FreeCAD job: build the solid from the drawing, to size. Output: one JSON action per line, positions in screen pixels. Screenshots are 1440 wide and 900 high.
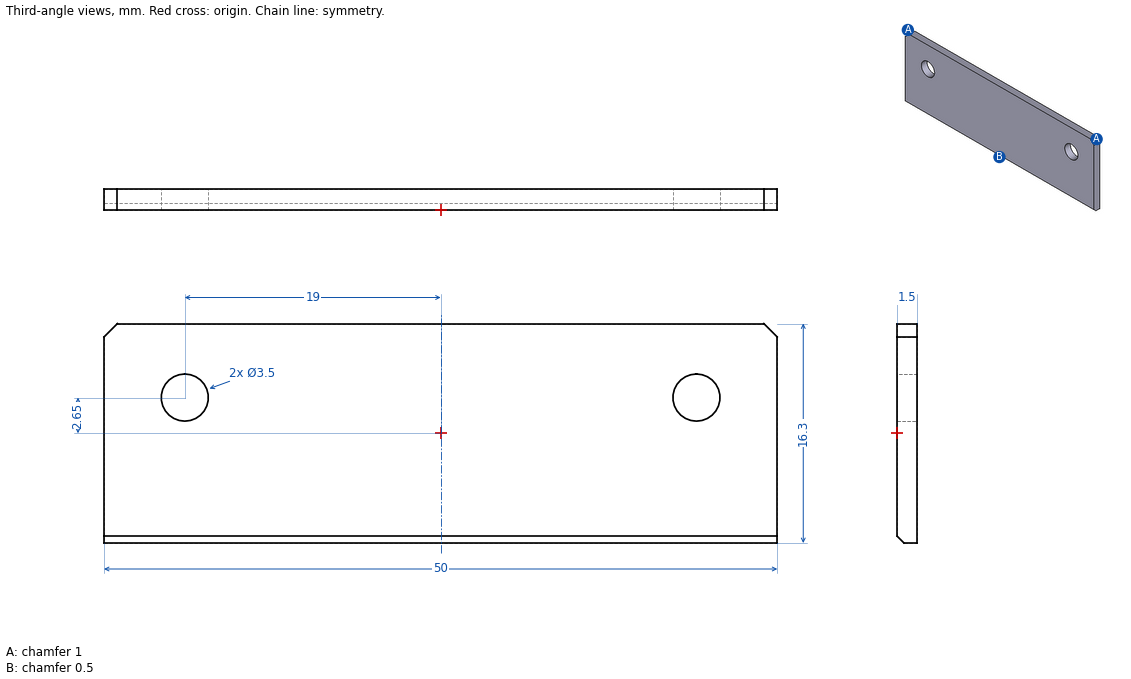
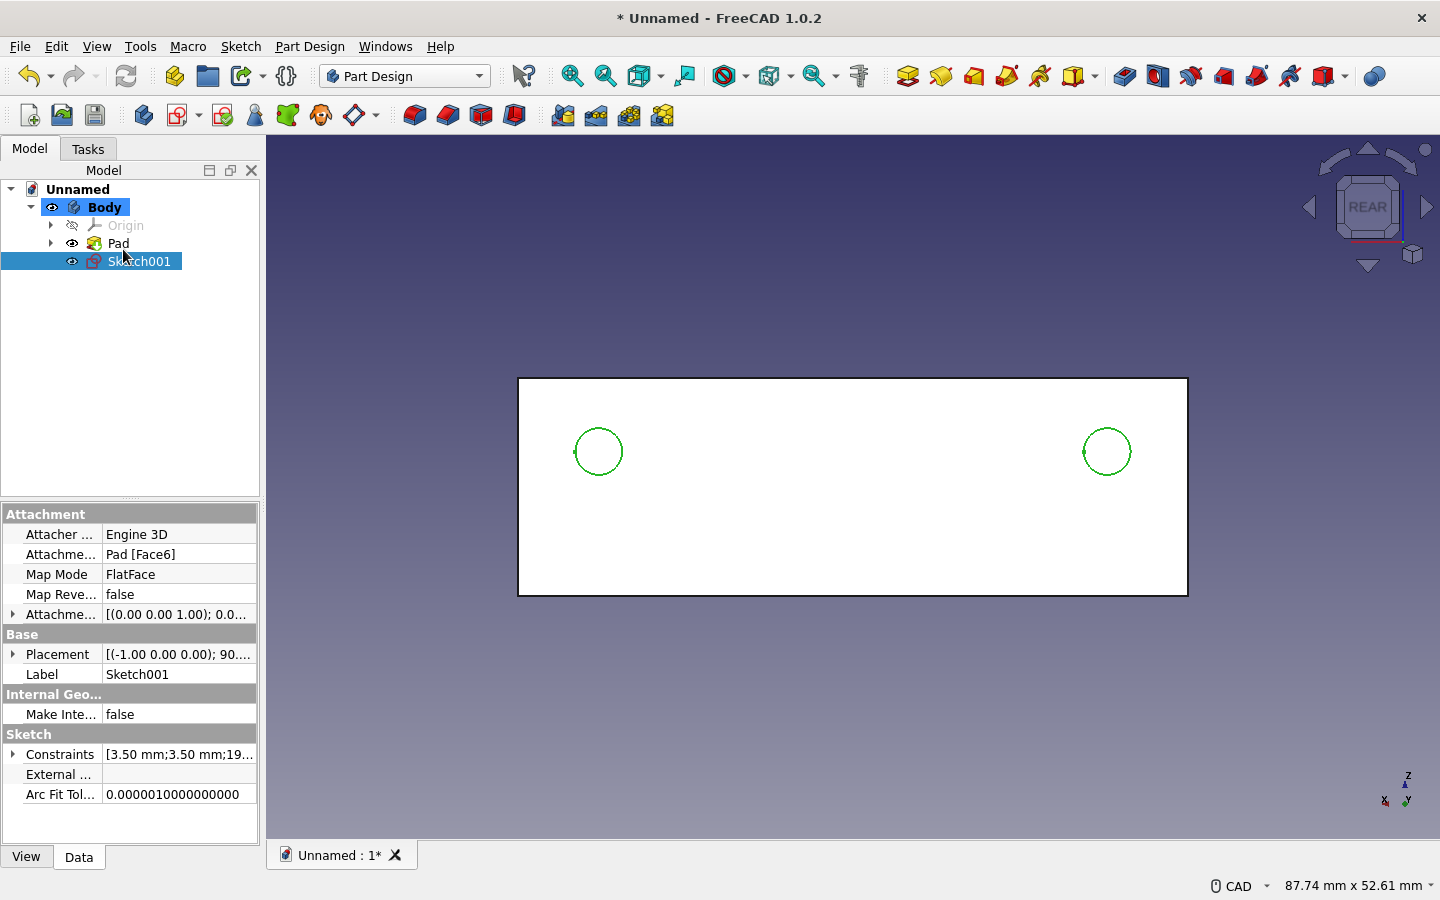
{"action": "left_click", "coordinate": [1125, 76]}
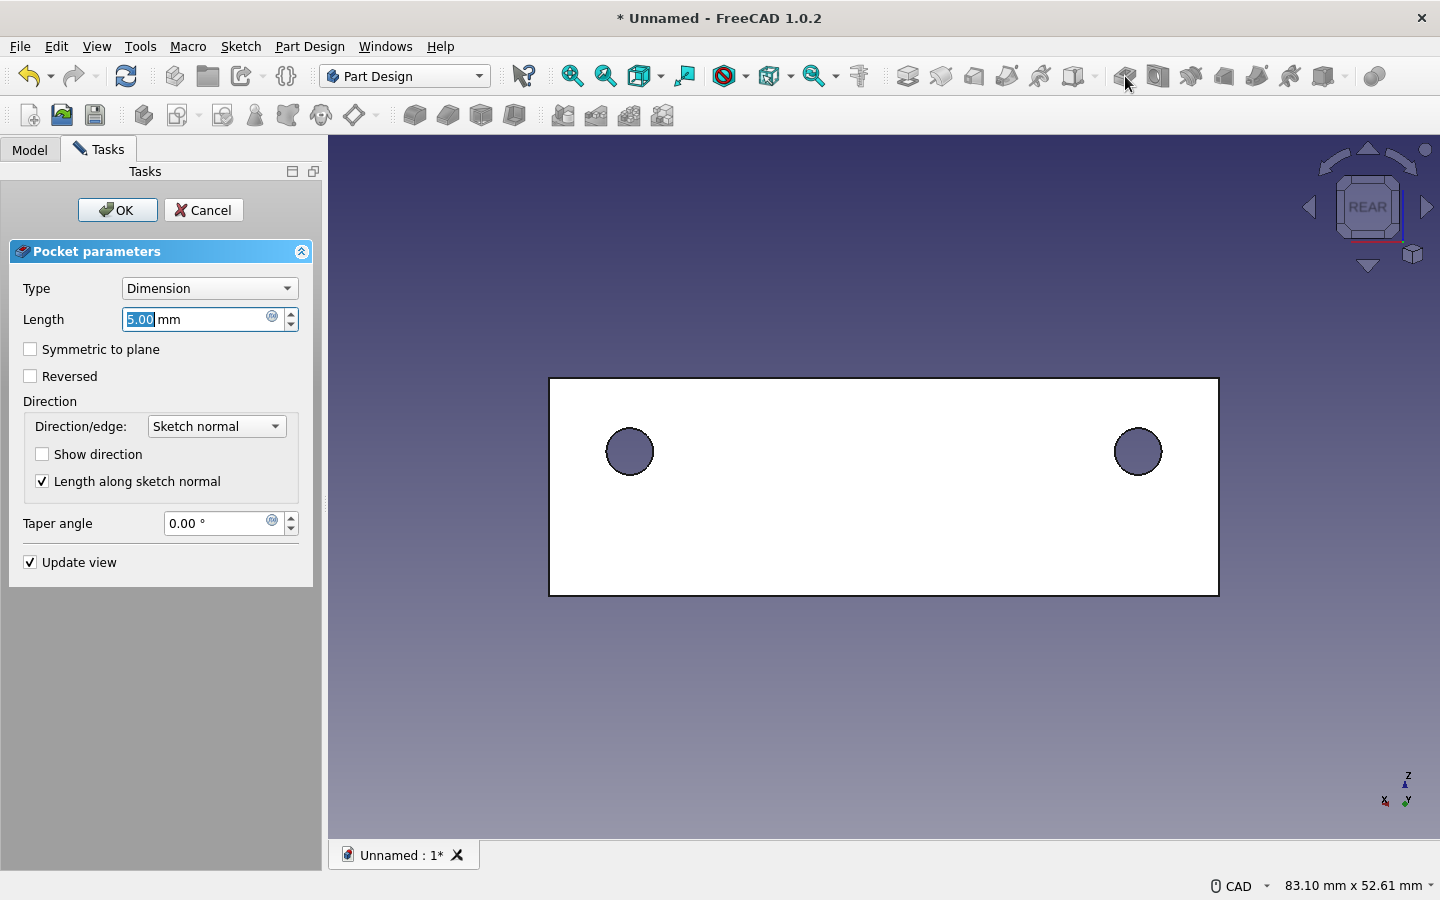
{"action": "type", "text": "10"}
{"action": "key", "text": "Tab"}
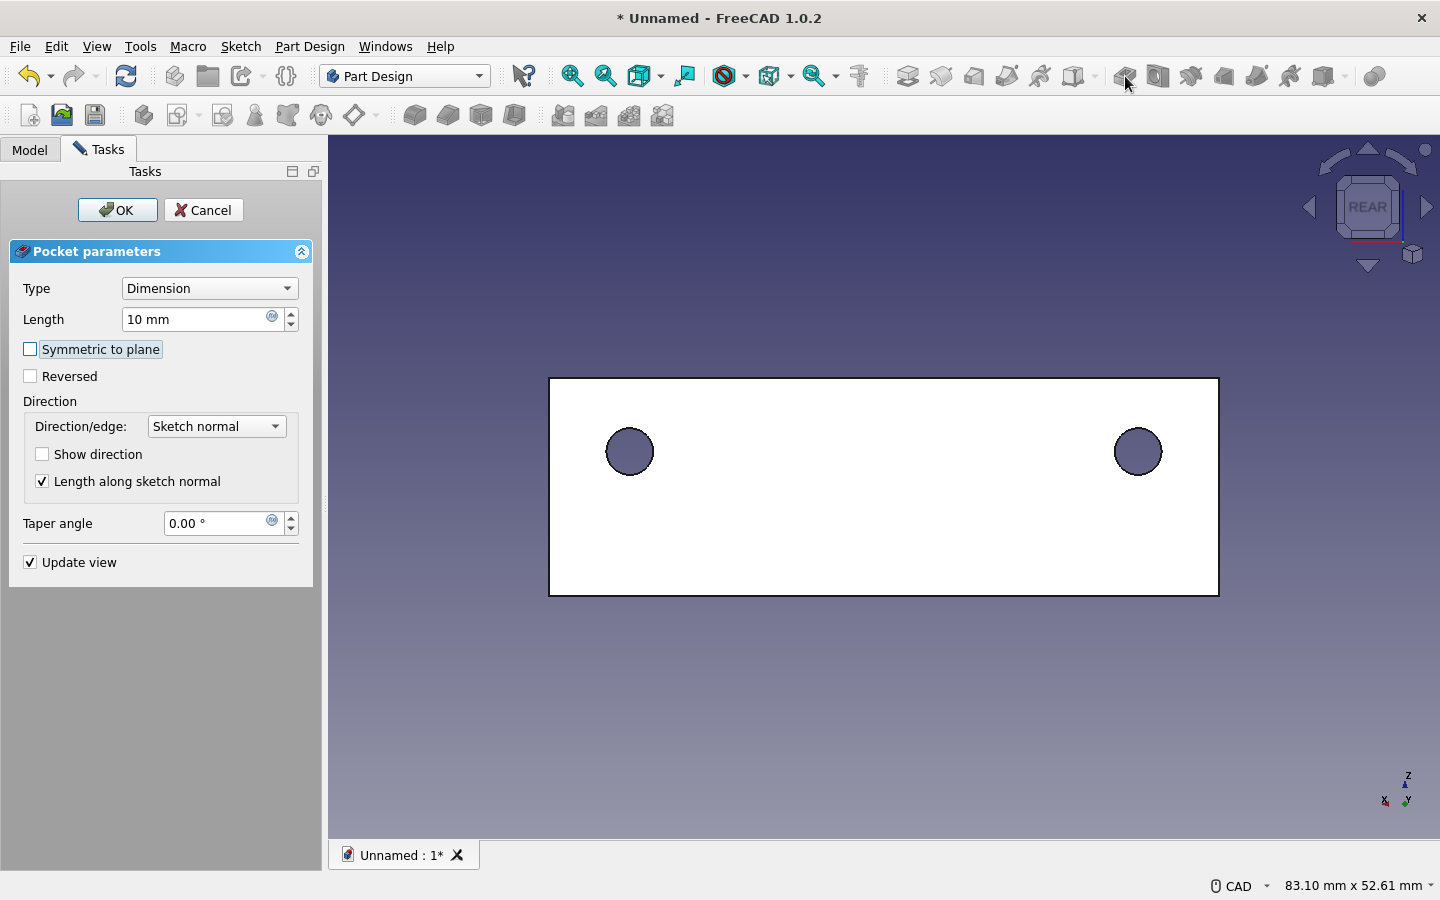
{"action": "left_click", "coordinate": [118, 210]}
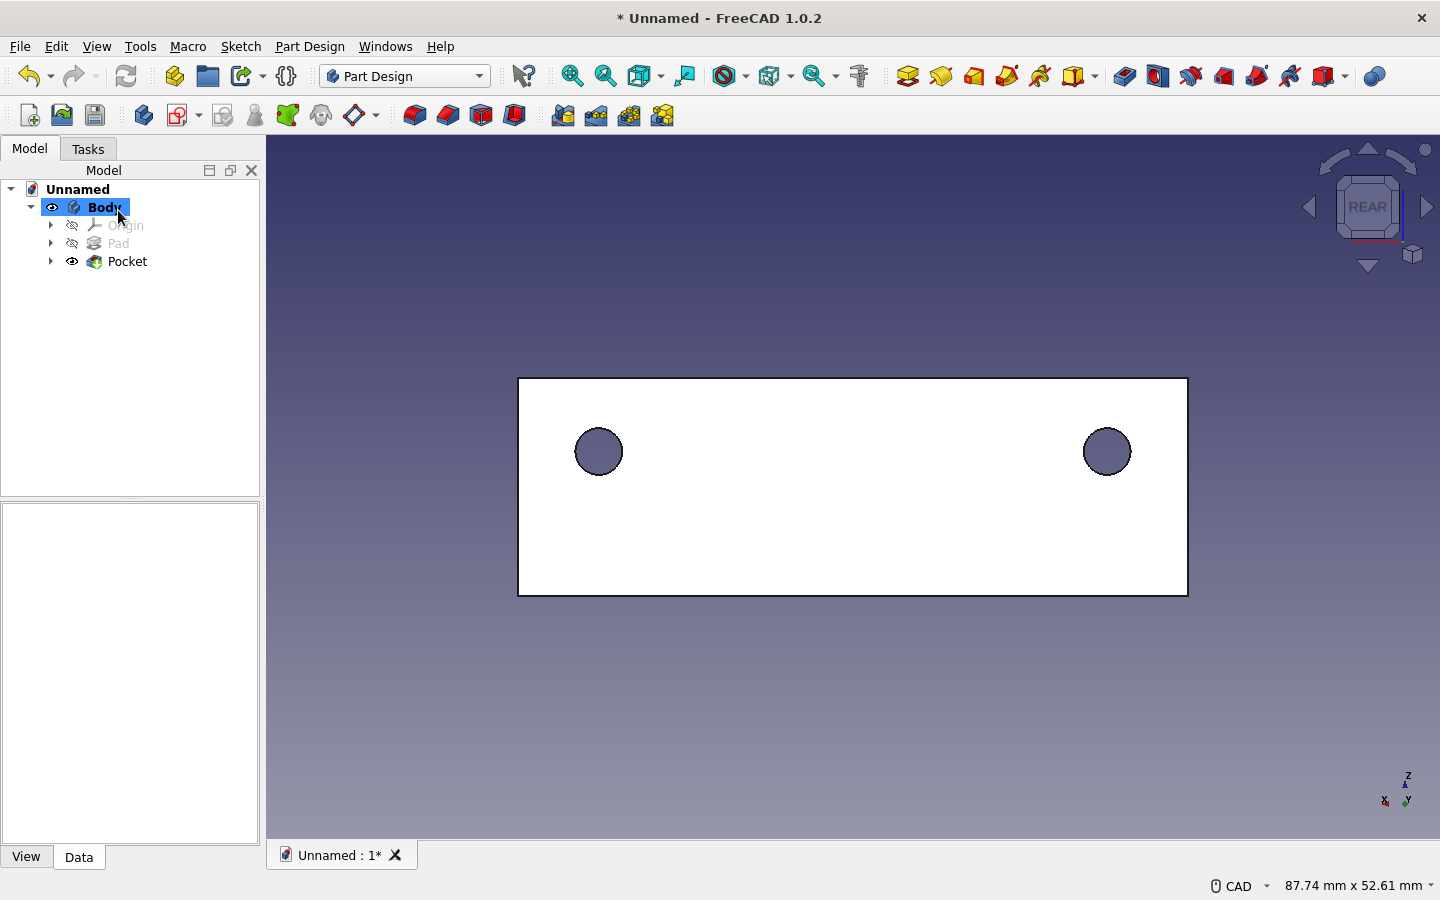
{"action": "scroll", "coordinate": [518, 377], "scroll_direction": "up", "scroll_amount": 4}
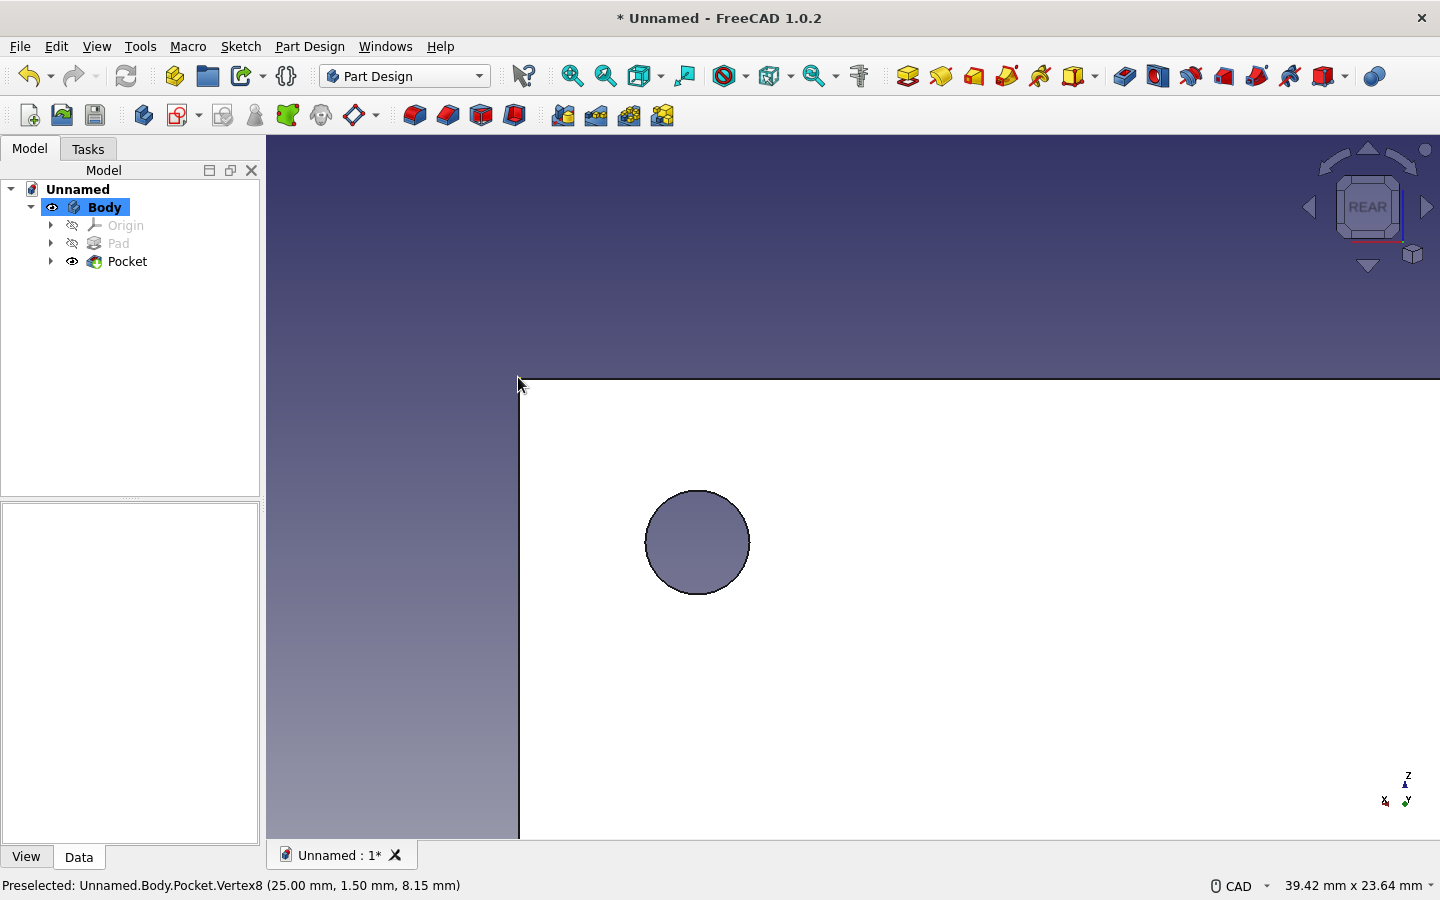
{"action": "key", "text": "v f"}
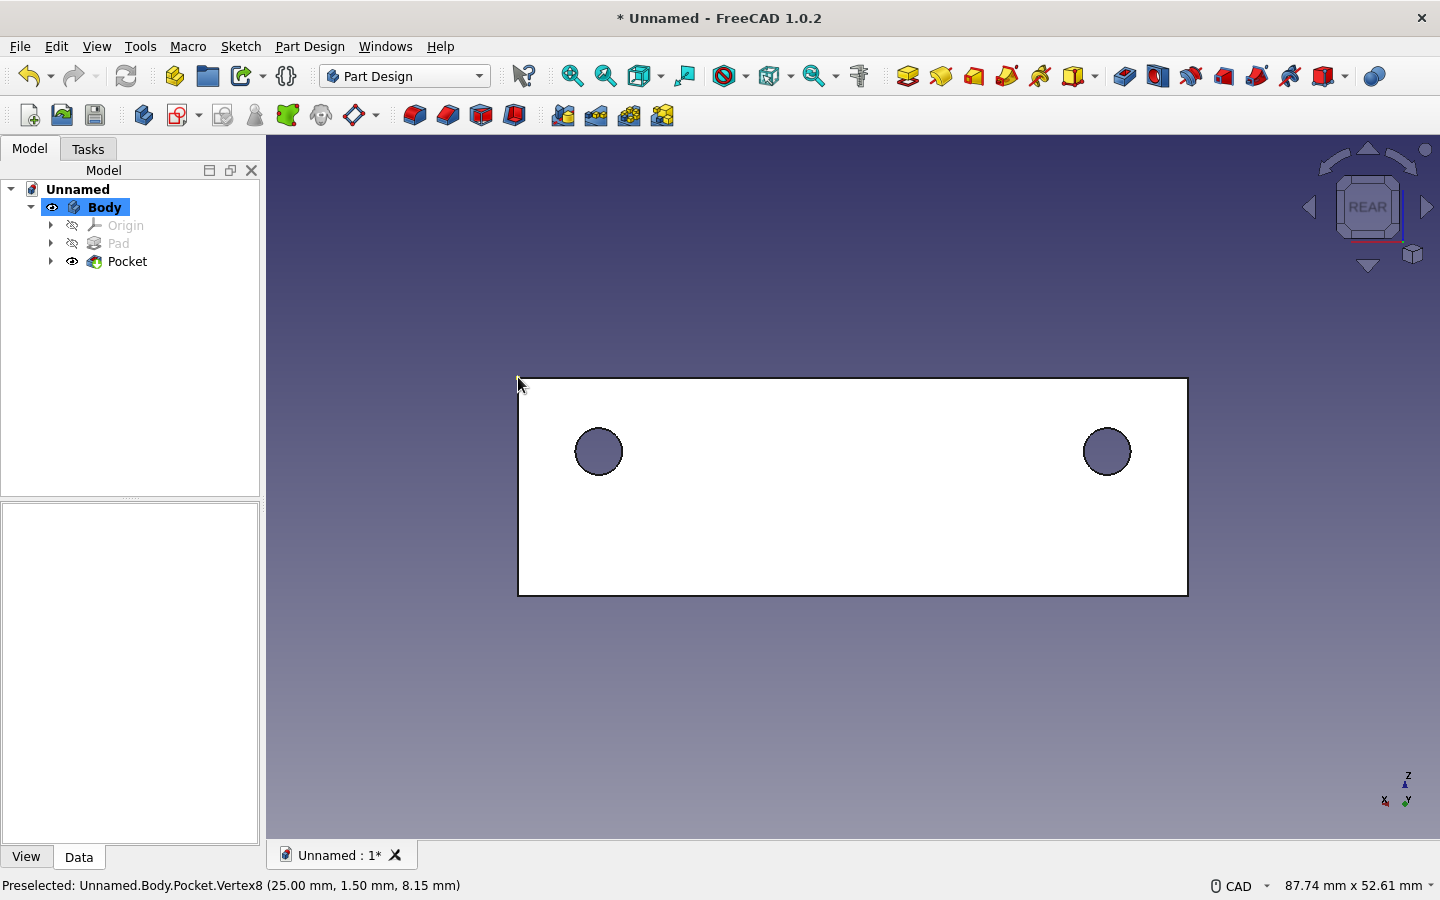
{"action": "key", "text": "0"}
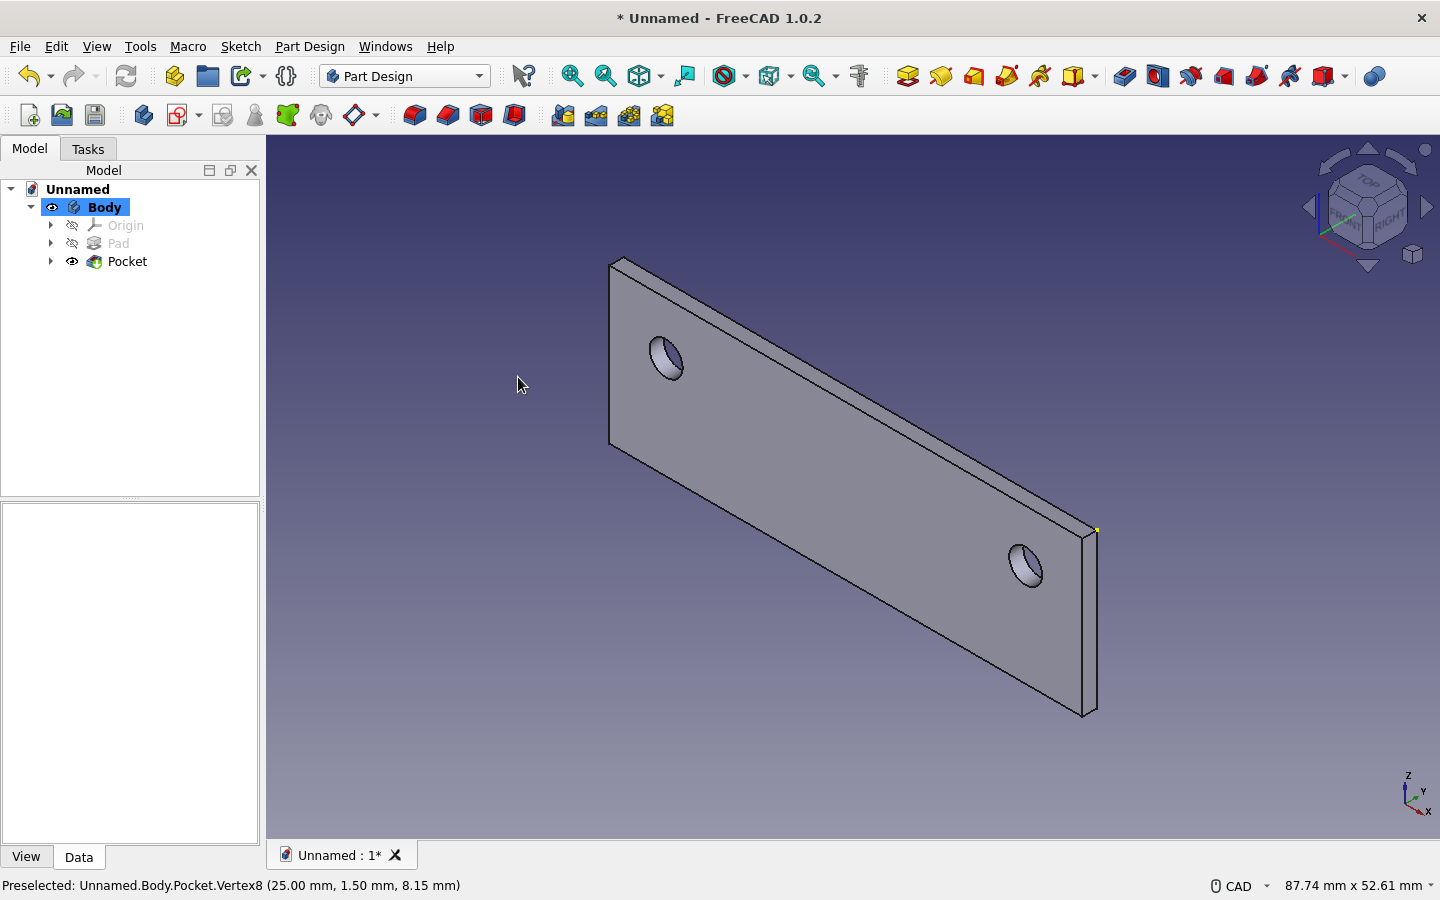
{"action": "left_click", "coordinate": [1090, 534]}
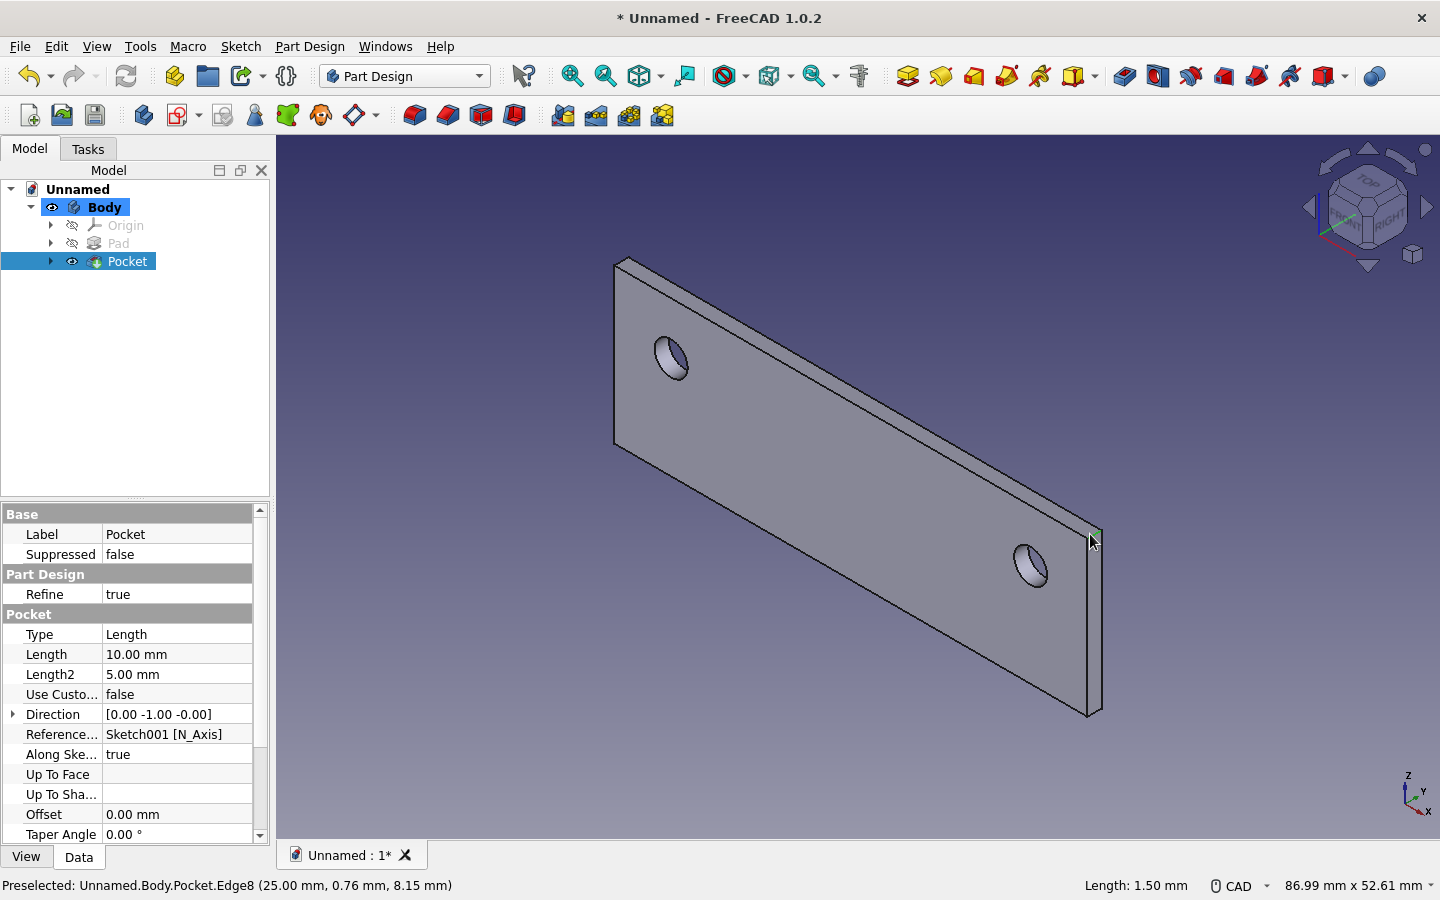
{"action": "scroll", "coordinate": [621, 260], "scroll_direction": "up", "scroll_amount": 4}